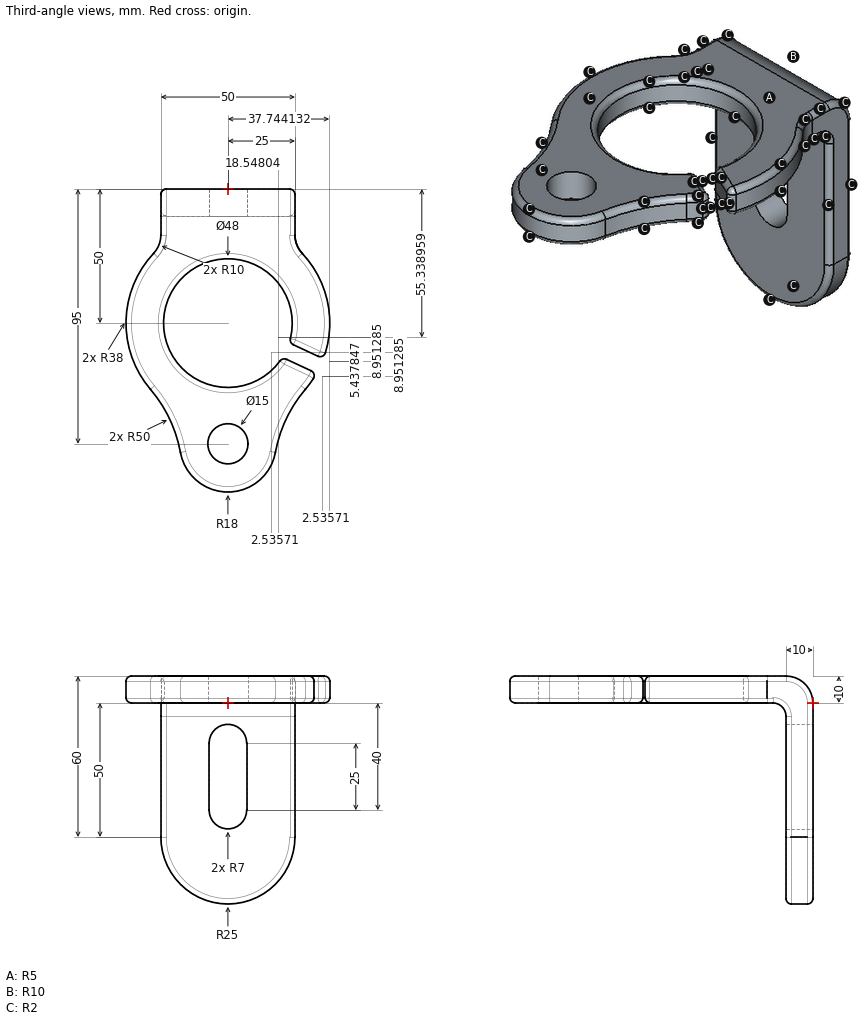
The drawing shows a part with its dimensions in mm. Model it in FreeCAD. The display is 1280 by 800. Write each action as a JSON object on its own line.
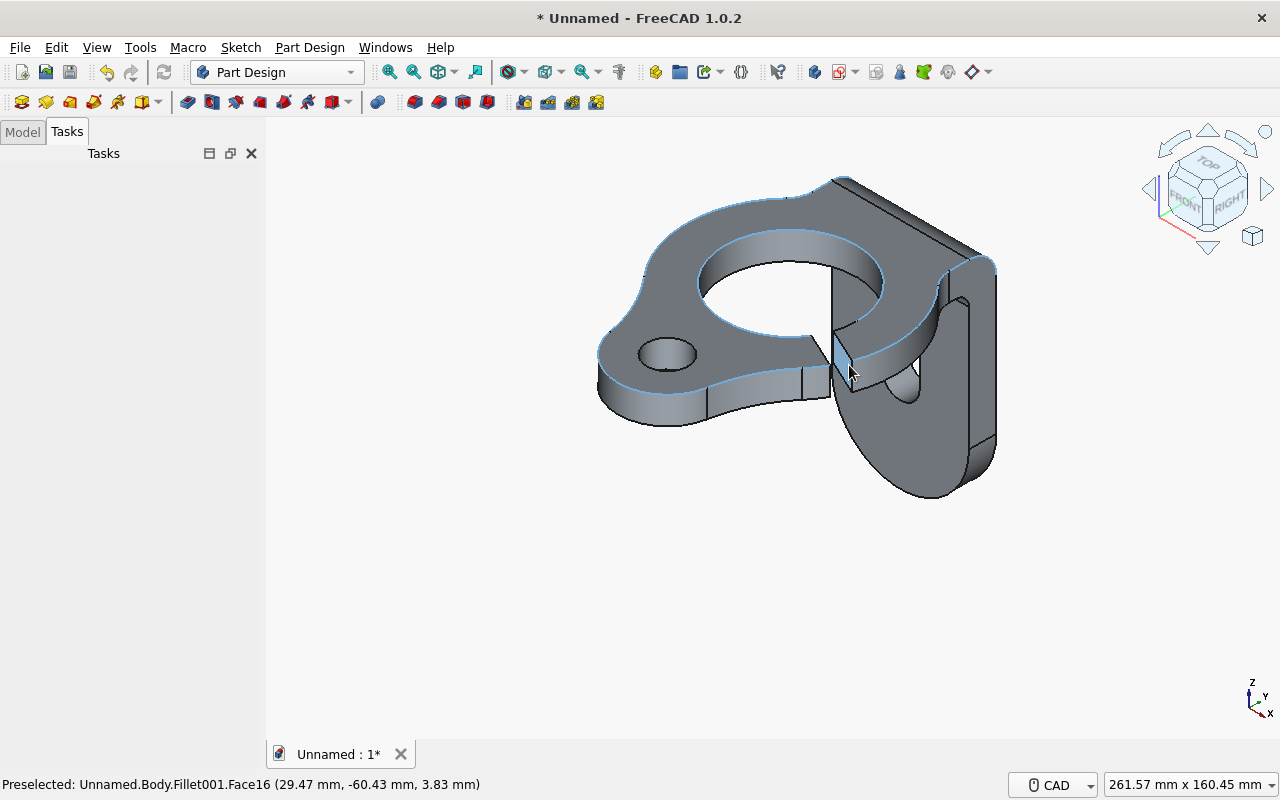
{"action": "left_click", "coordinate": [969, 377], "text": "ctrl"}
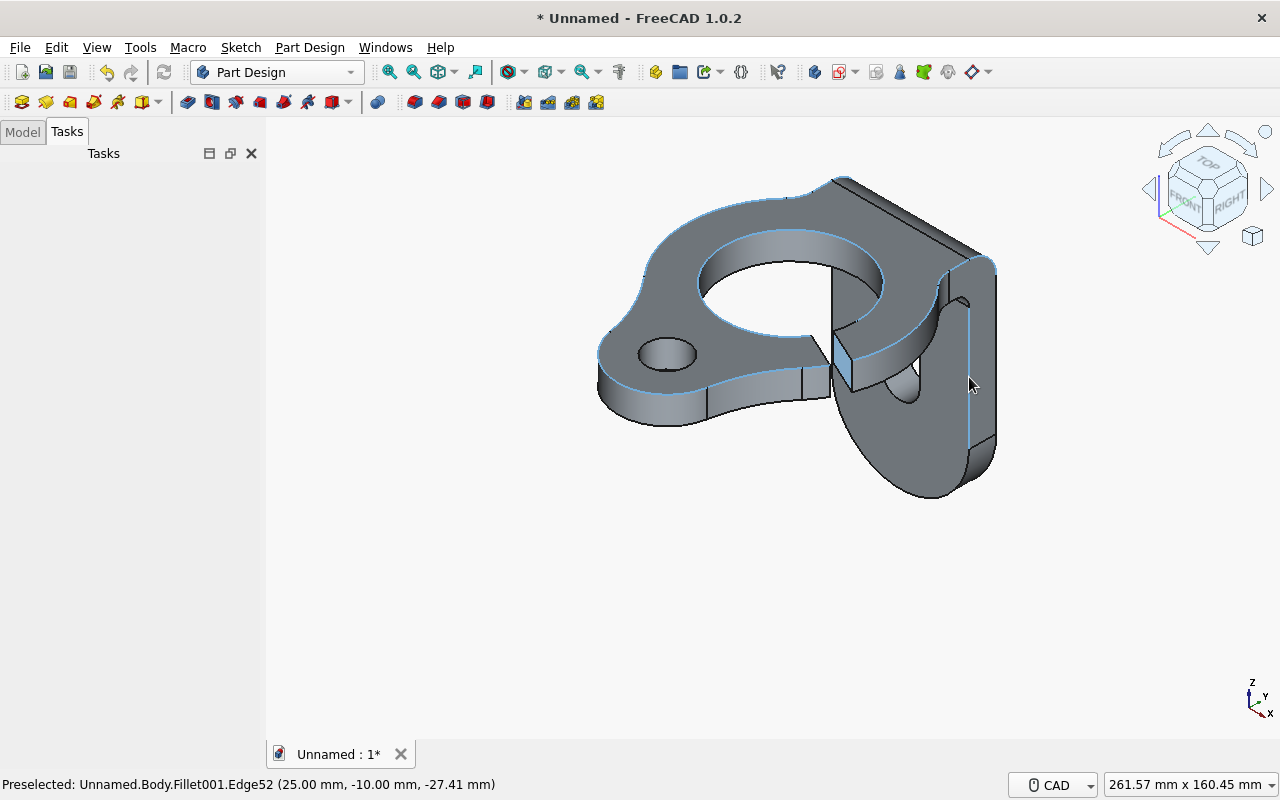
{"action": "left_click", "coordinate": [965, 297], "text": "ctrl"}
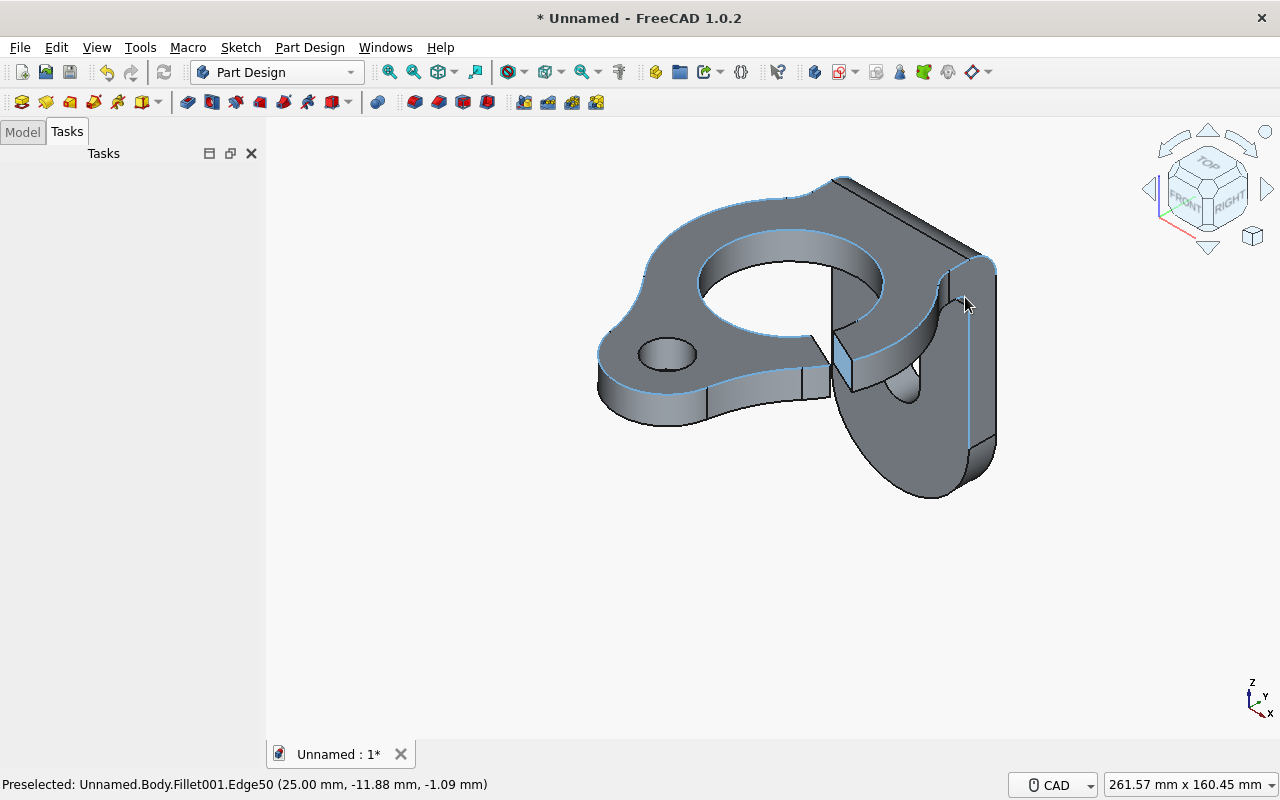
{"action": "left_click", "coordinate": [992, 459], "text": "ctrl"}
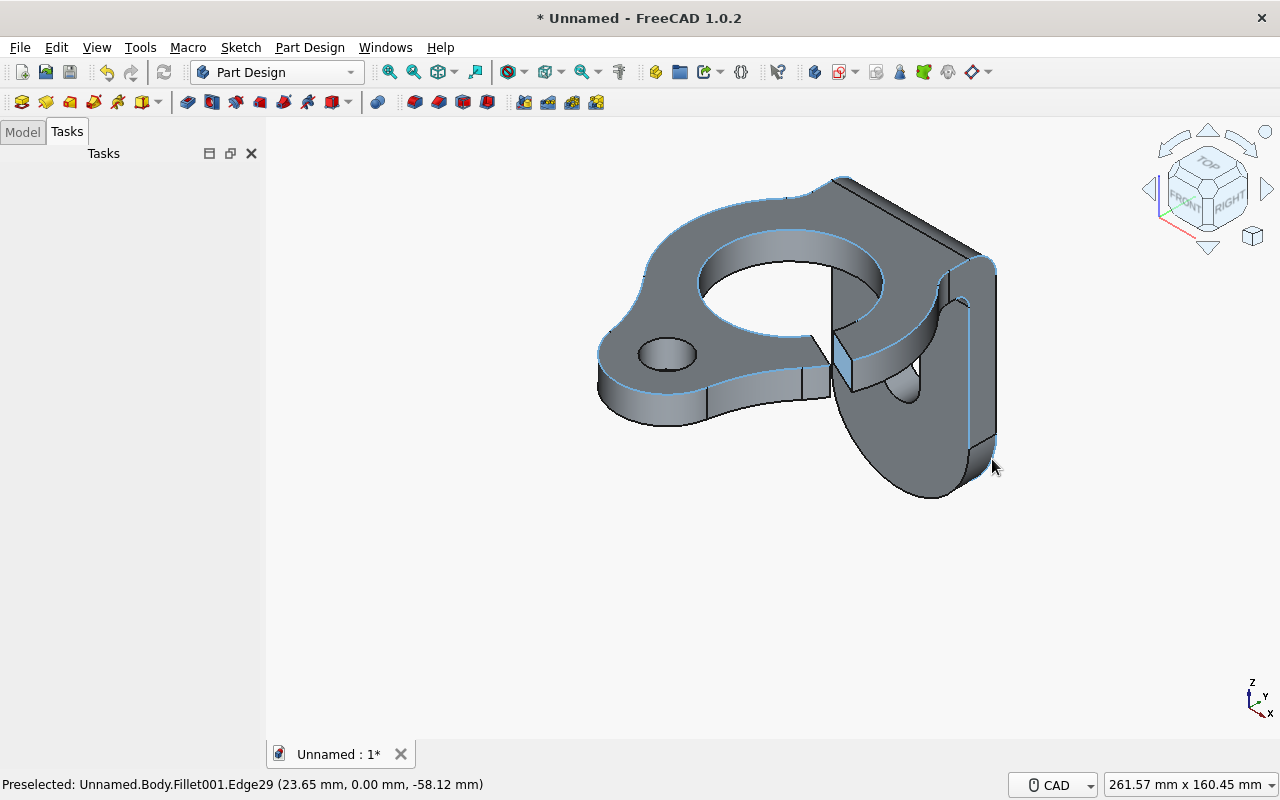
{"action": "left_click", "coordinate": [956, 487], "text": "ctrl"}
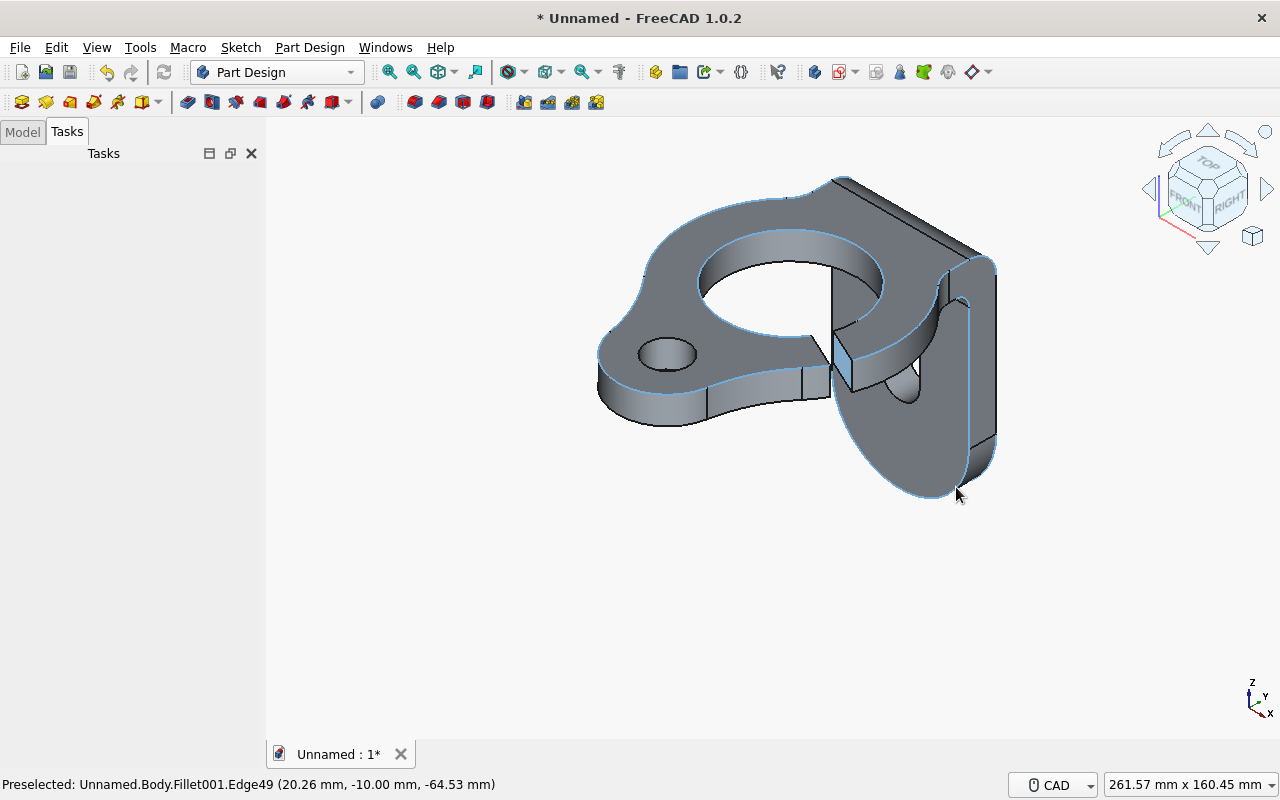
{"action": "key", "text": "2"}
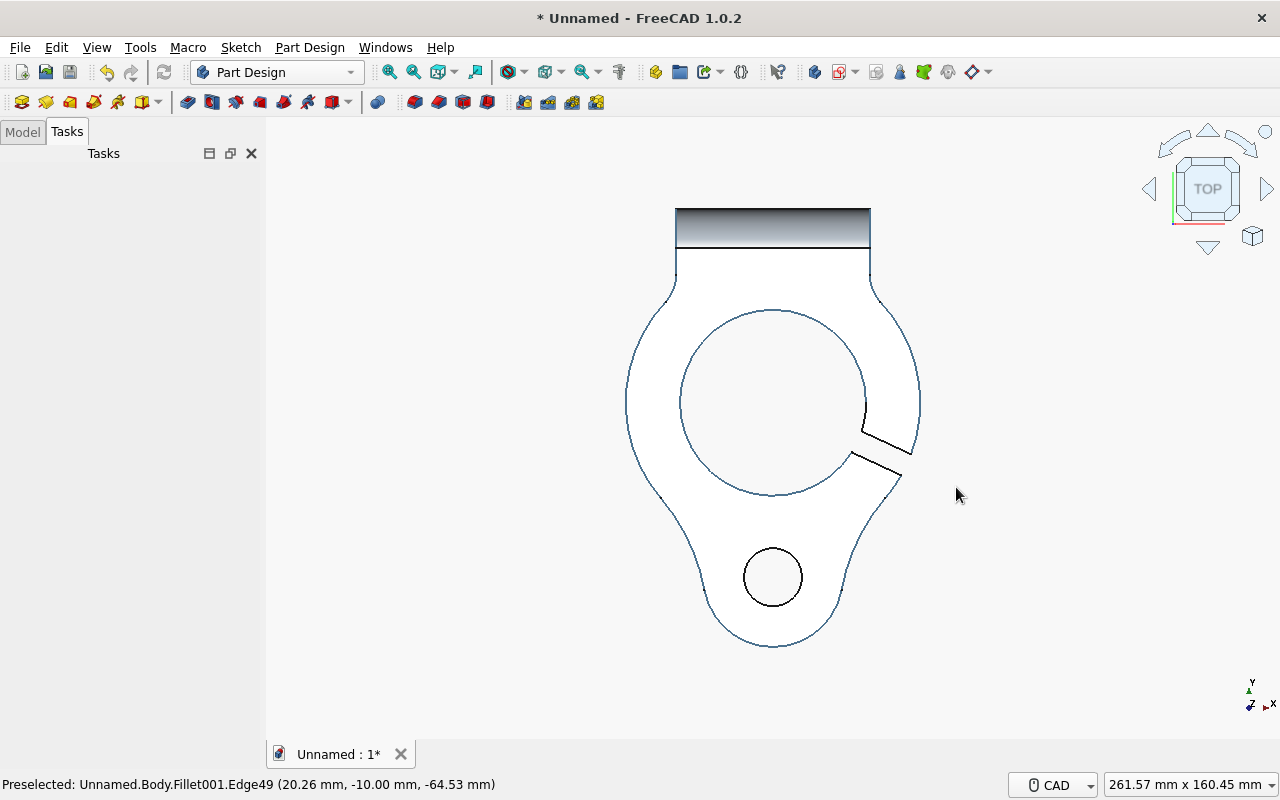
{"action": "key", "text": "1"}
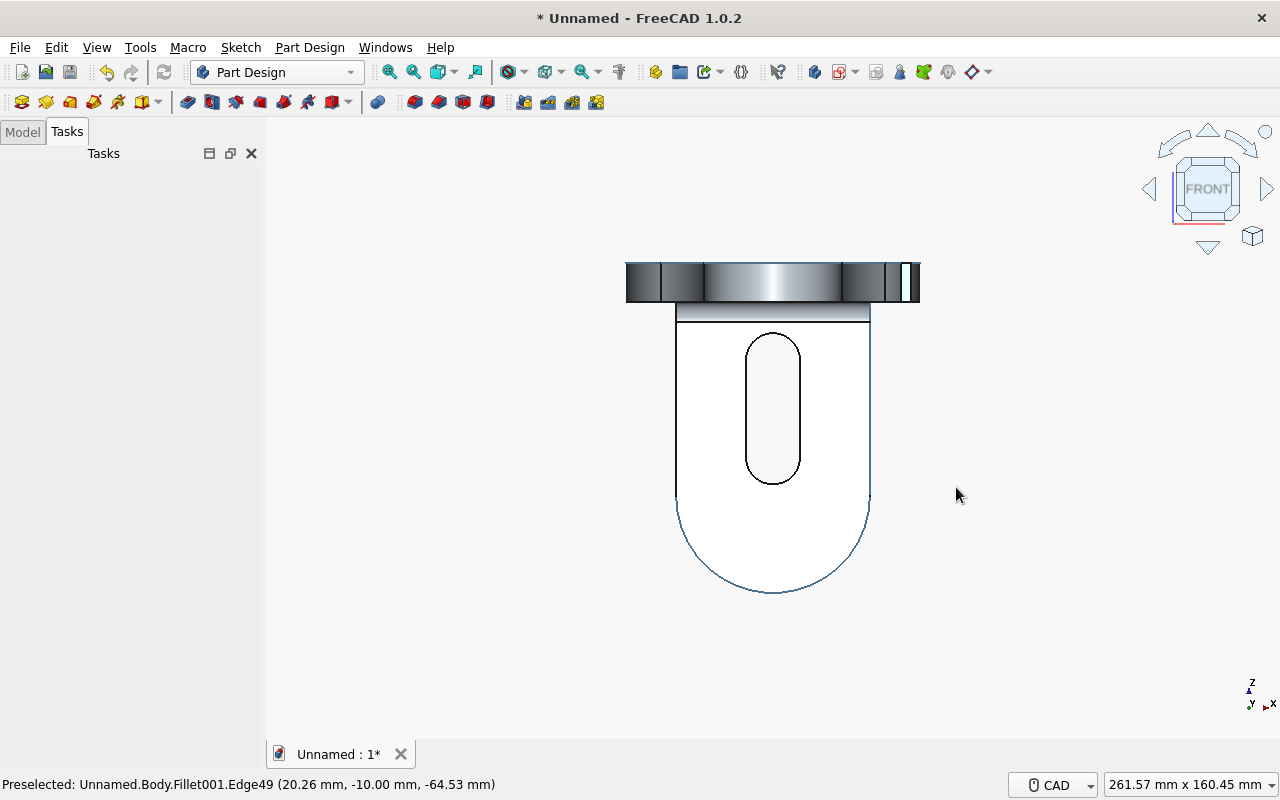
{"action": "left_click", "coordinate": [628, 301], "text": "ctrl"}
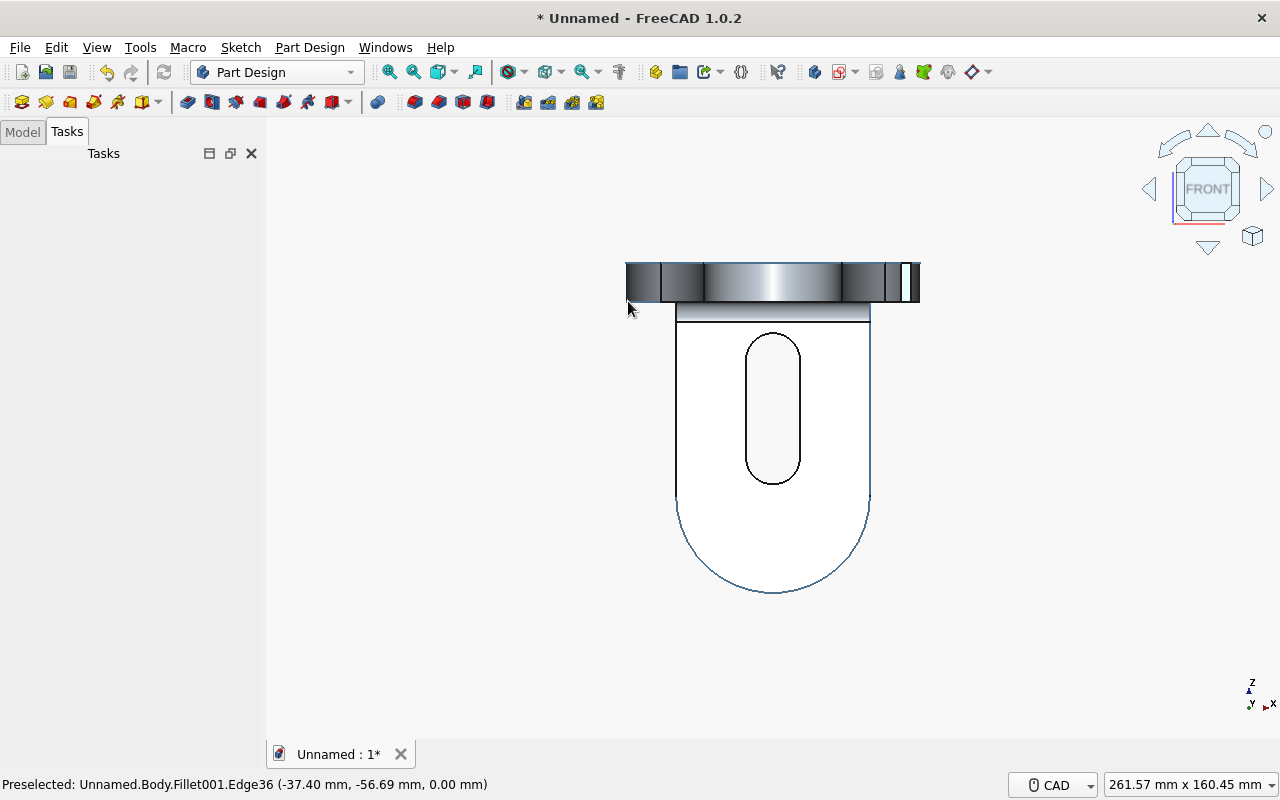
{"action": "left_click", "coordinate": [676, 309], "text": "ctrl"}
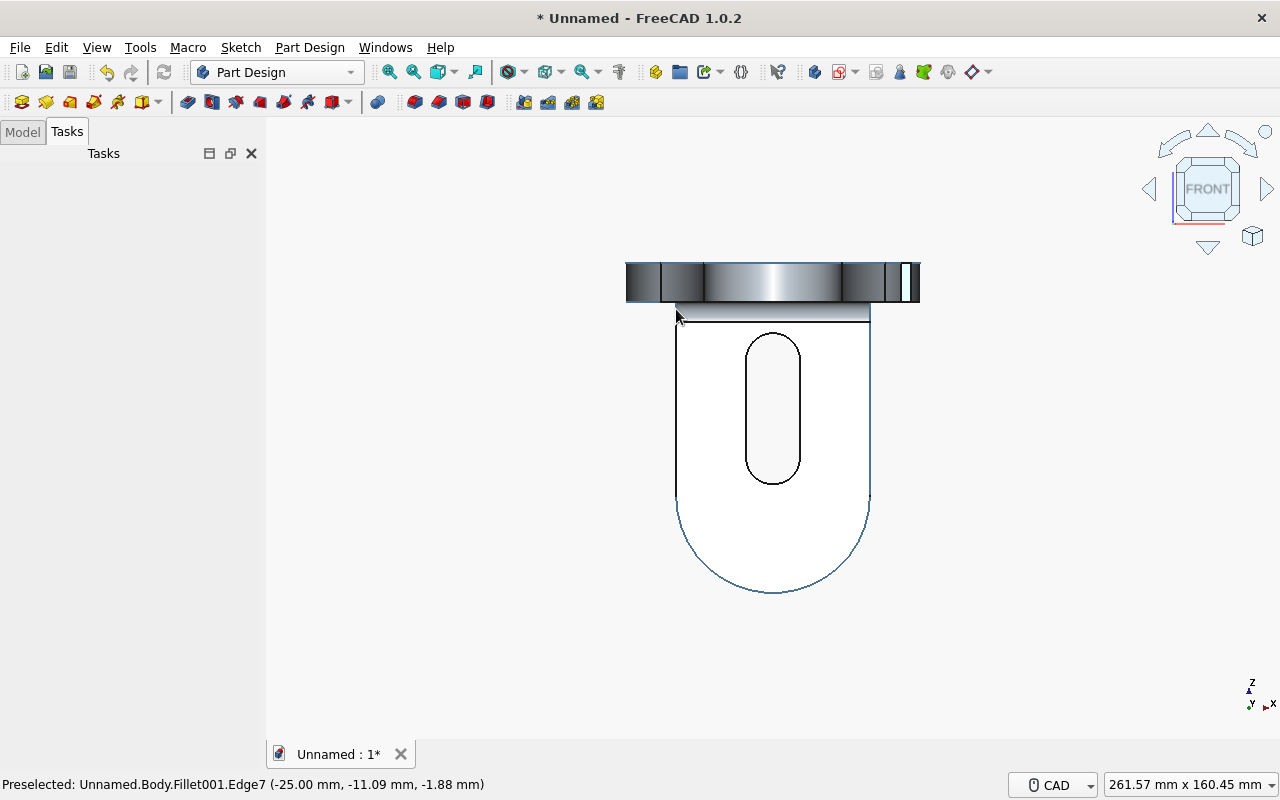
{"action": "left_click", "coordinate": [894, 301], "text": "ctrl"}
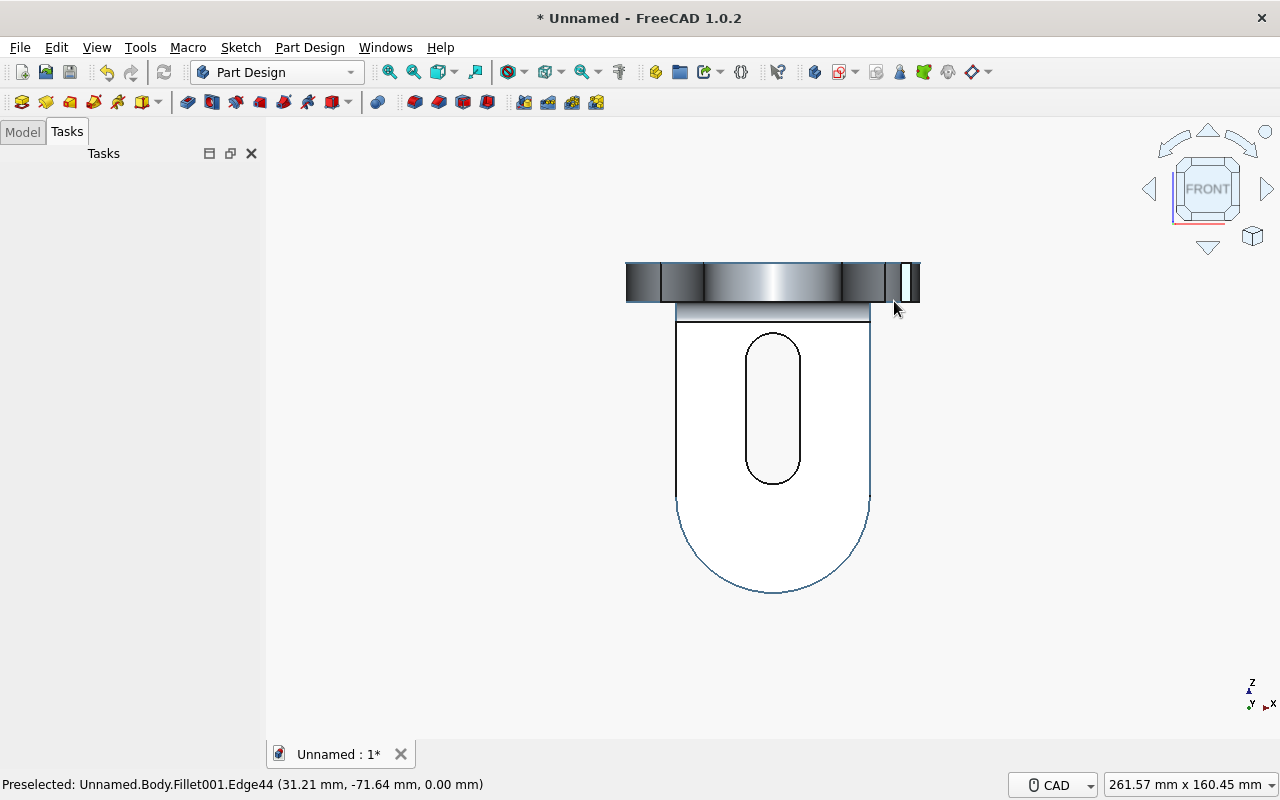
{"action": "left_click", "coordinate": [857, 301], "text": "ctrl"}